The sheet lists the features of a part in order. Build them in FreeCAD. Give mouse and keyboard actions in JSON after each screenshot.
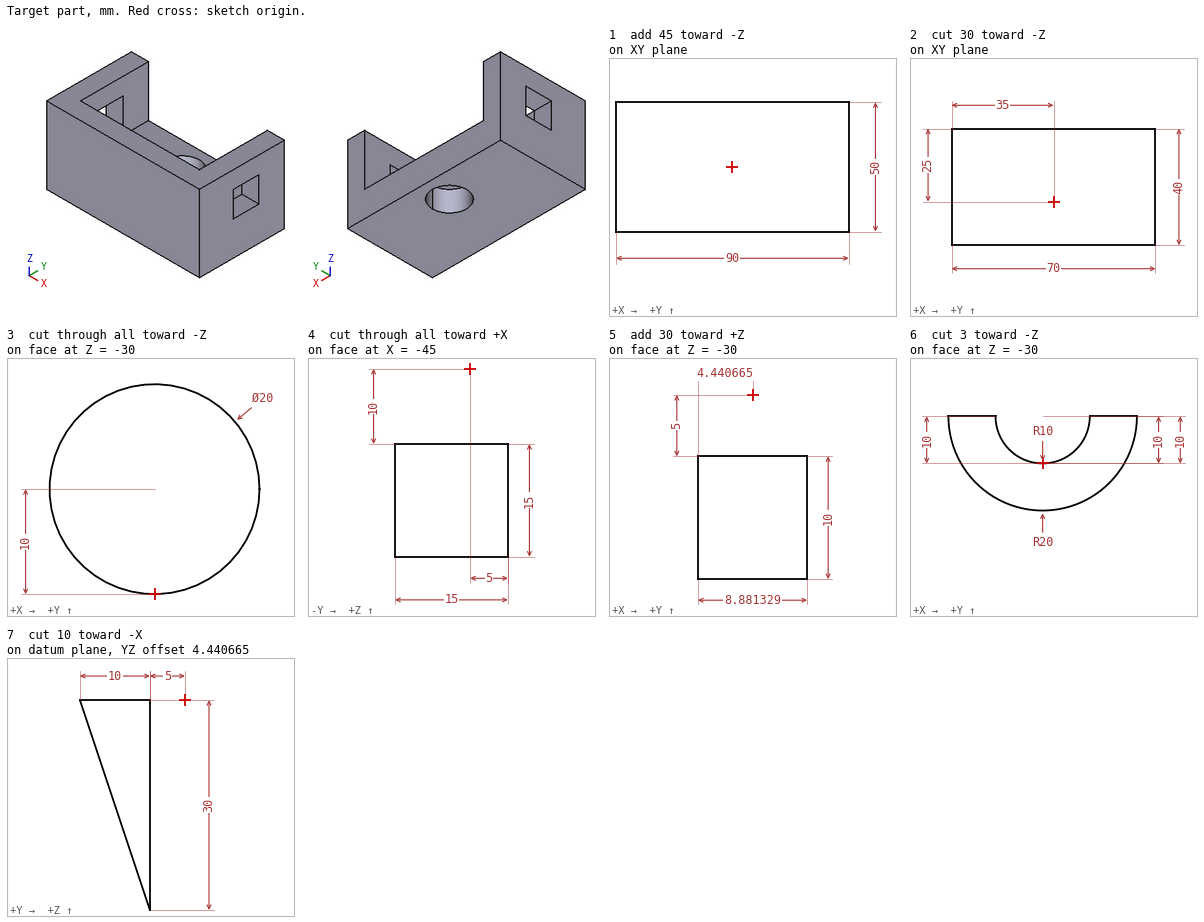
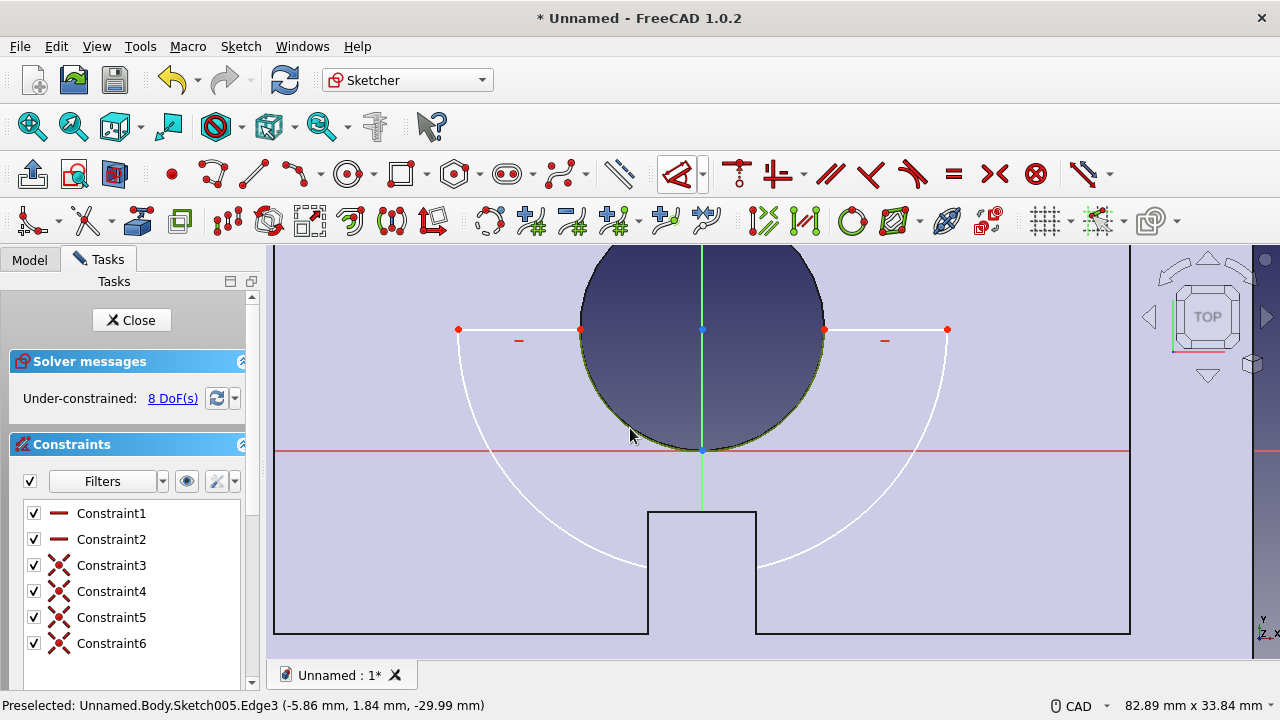
{"action": "left_click", "coordinate": [559, 527]}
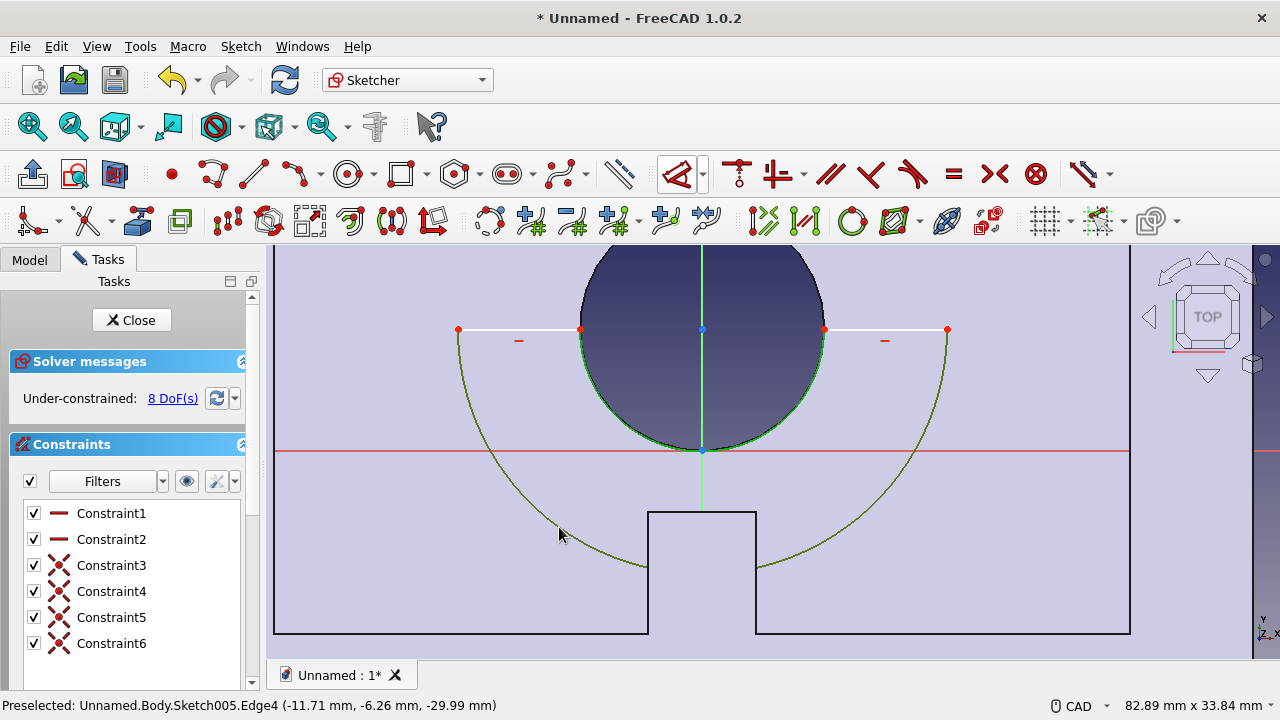
{"action": "key", "text": "c"}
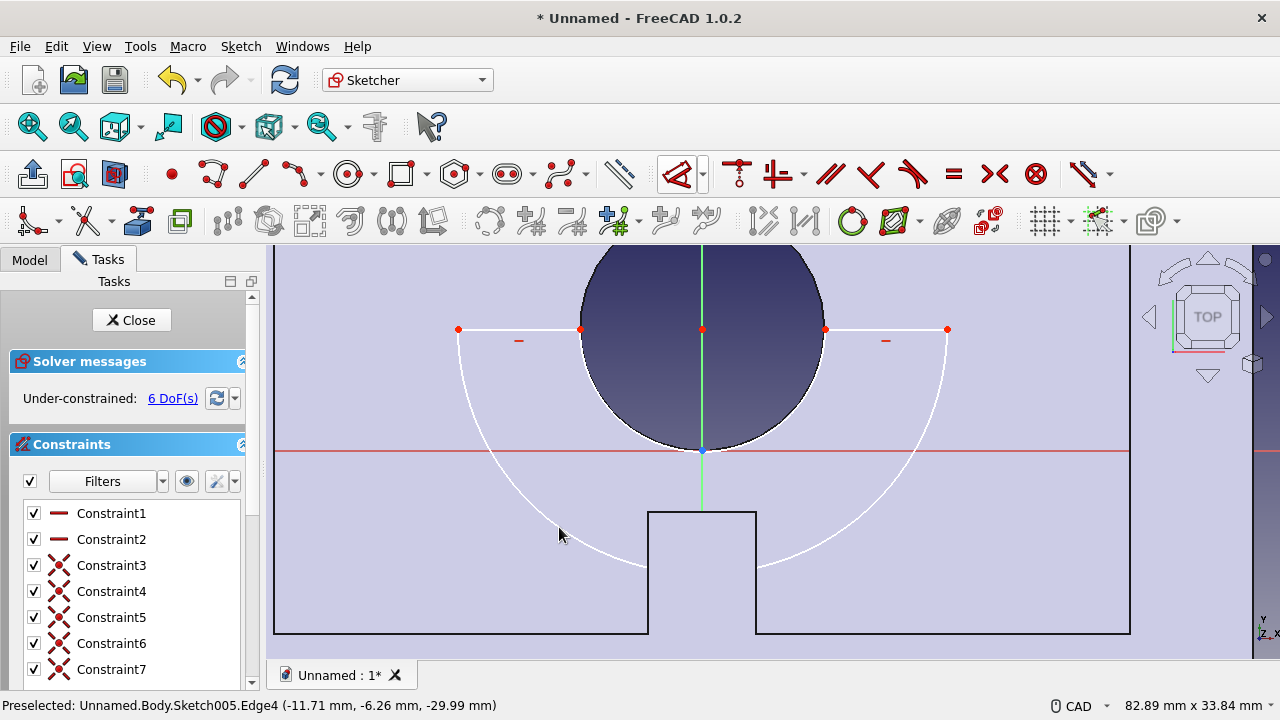
{"action": "left_click", "coordinate": [703, 329]}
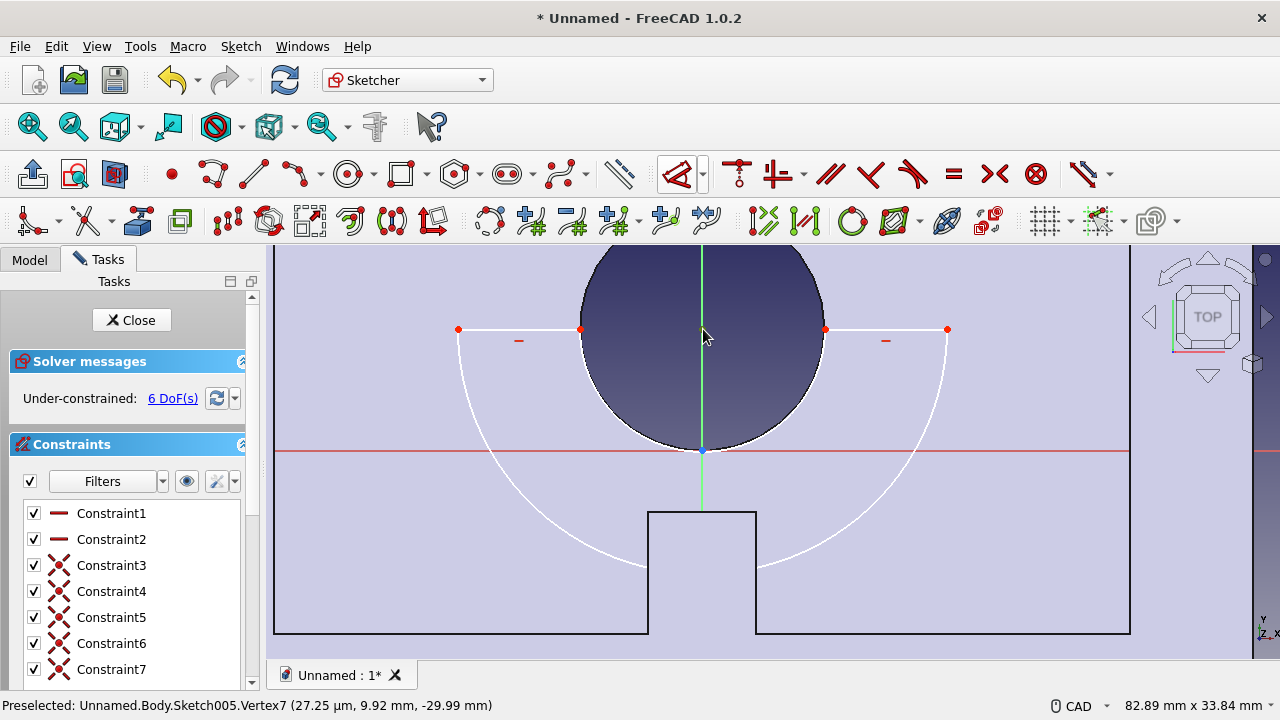
{"action": "left_click", "coordinate": [702, 605]}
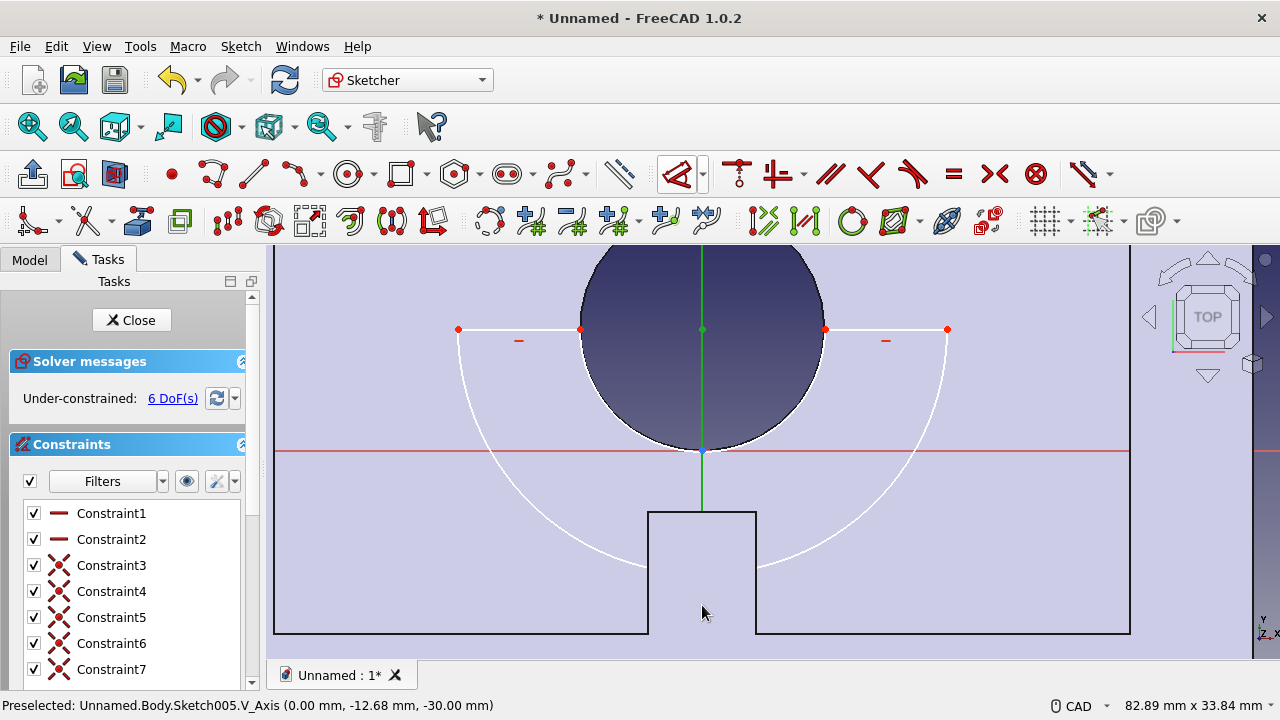
{"action": "key", "text": "c"}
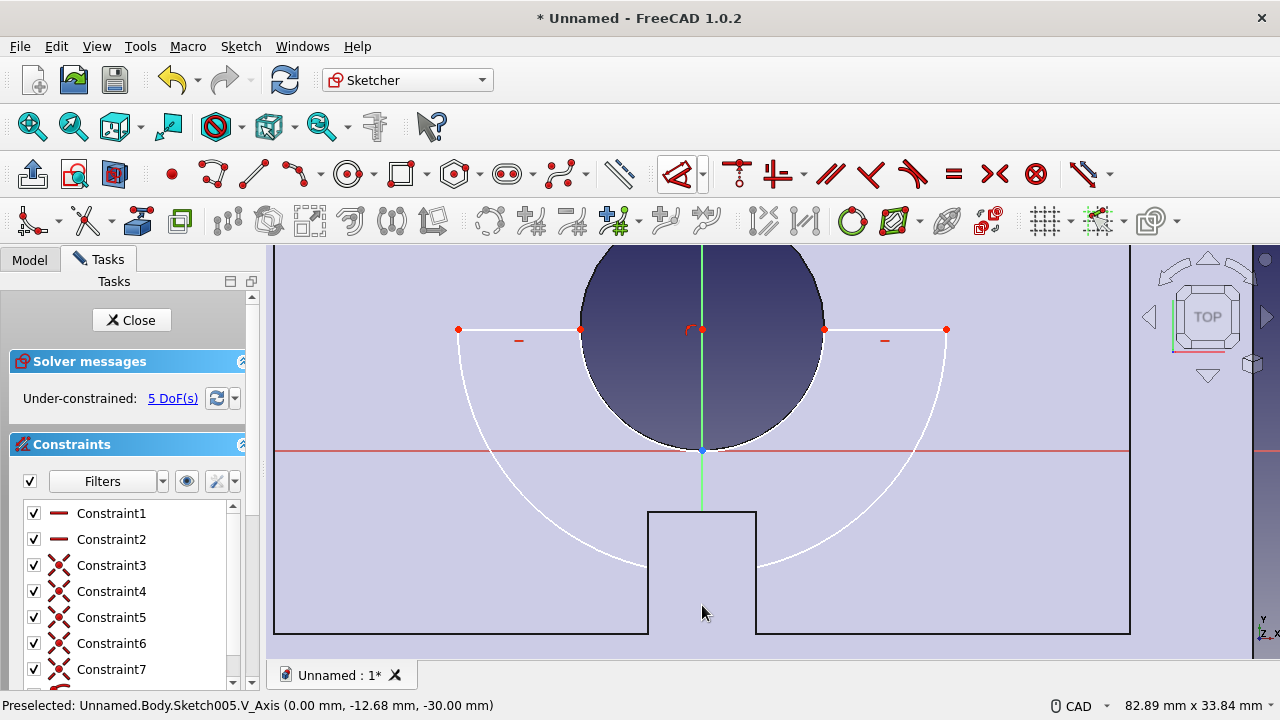
{"action": "left_click", "coordinate": [631, 428]}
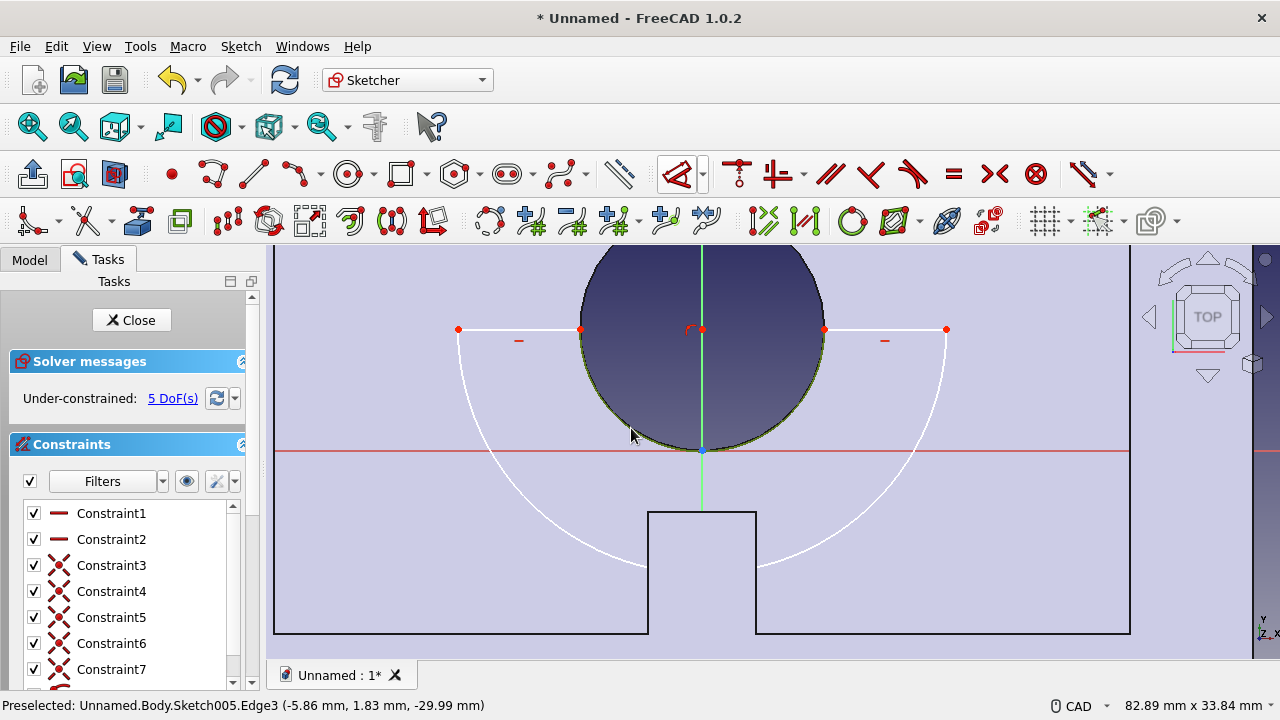
{"action": "key", "text": "k r"}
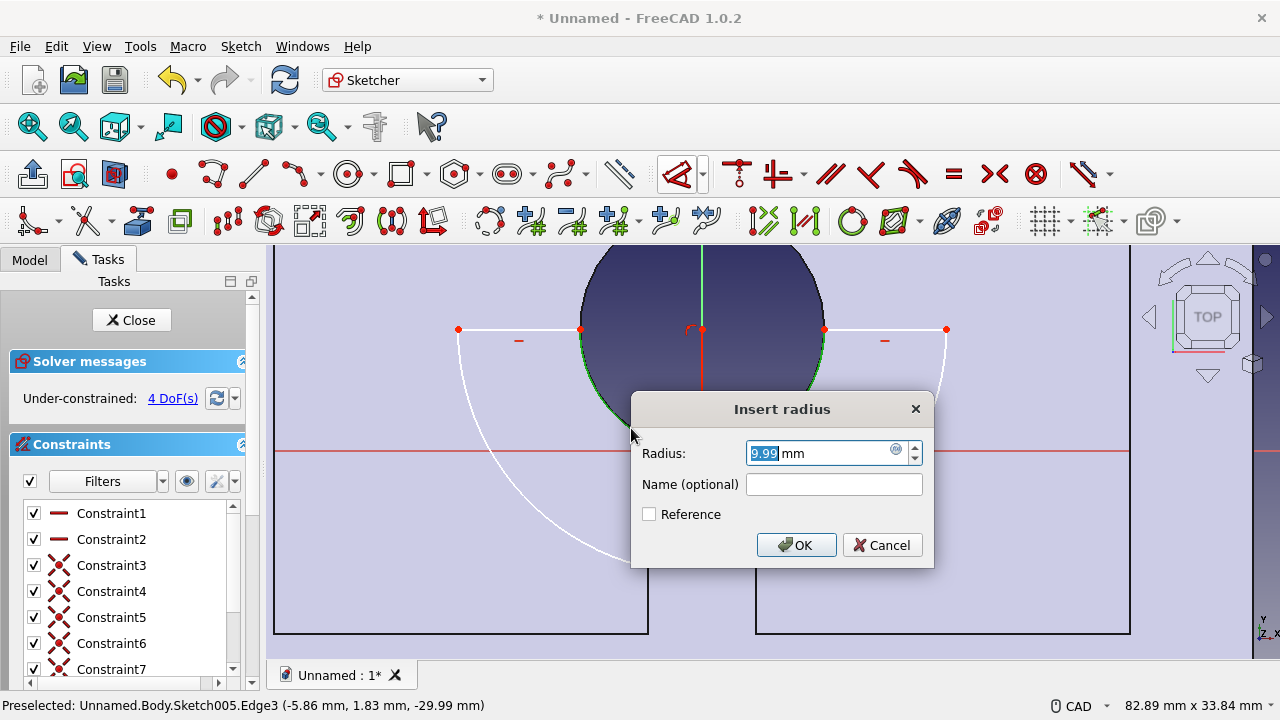
{"action": "type", "text": "10"}
{"action": "key", "text": "Return"}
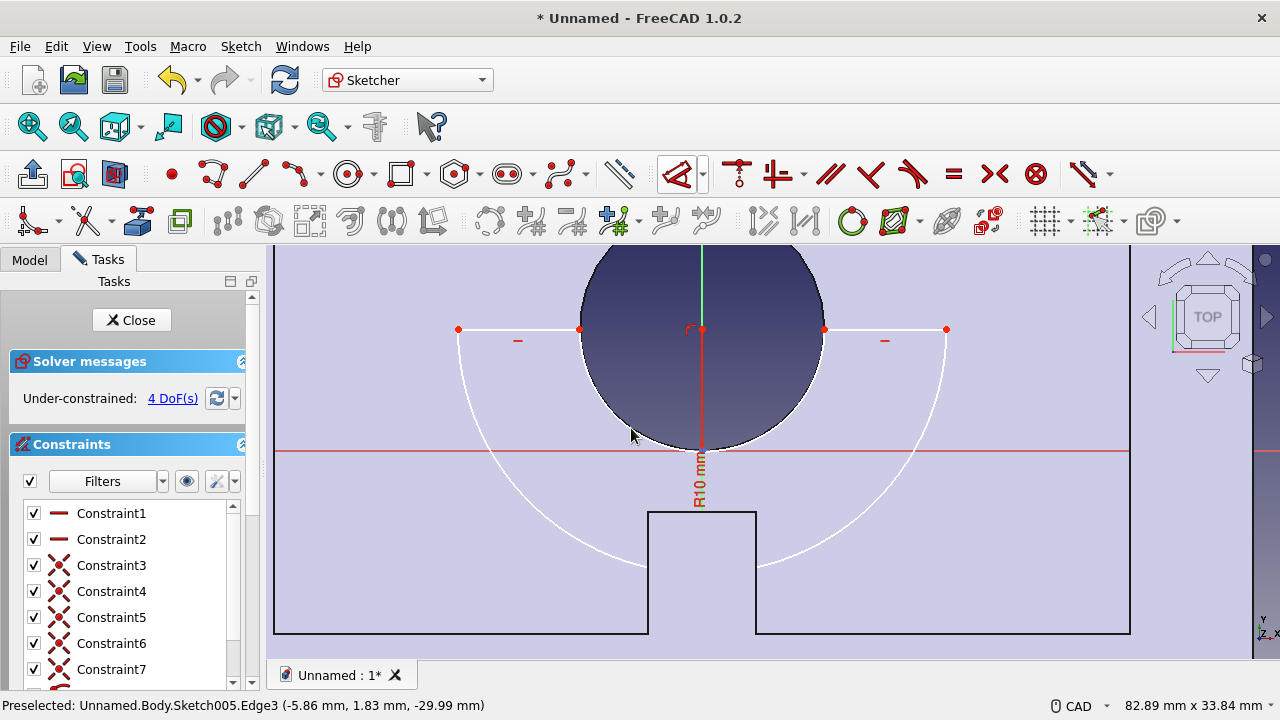
{"action": "left_click", "coordinate": [559, 527]}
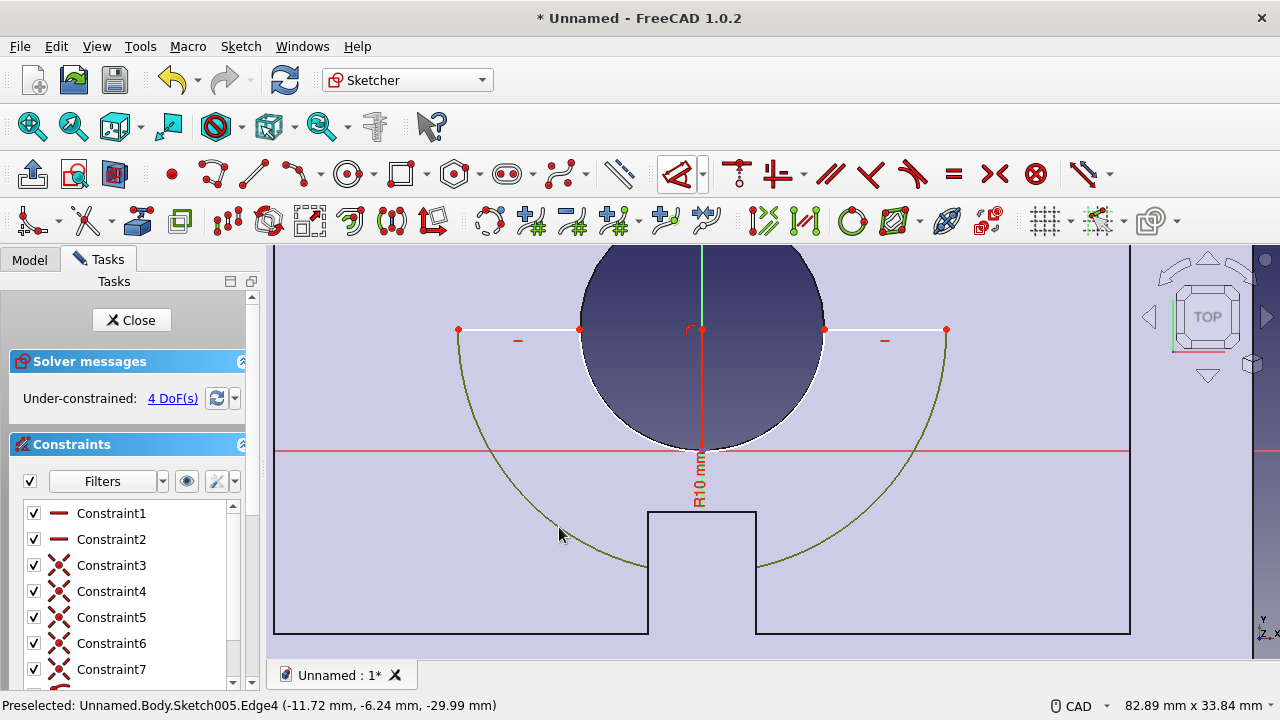
{"action": "key", "text": "k r"}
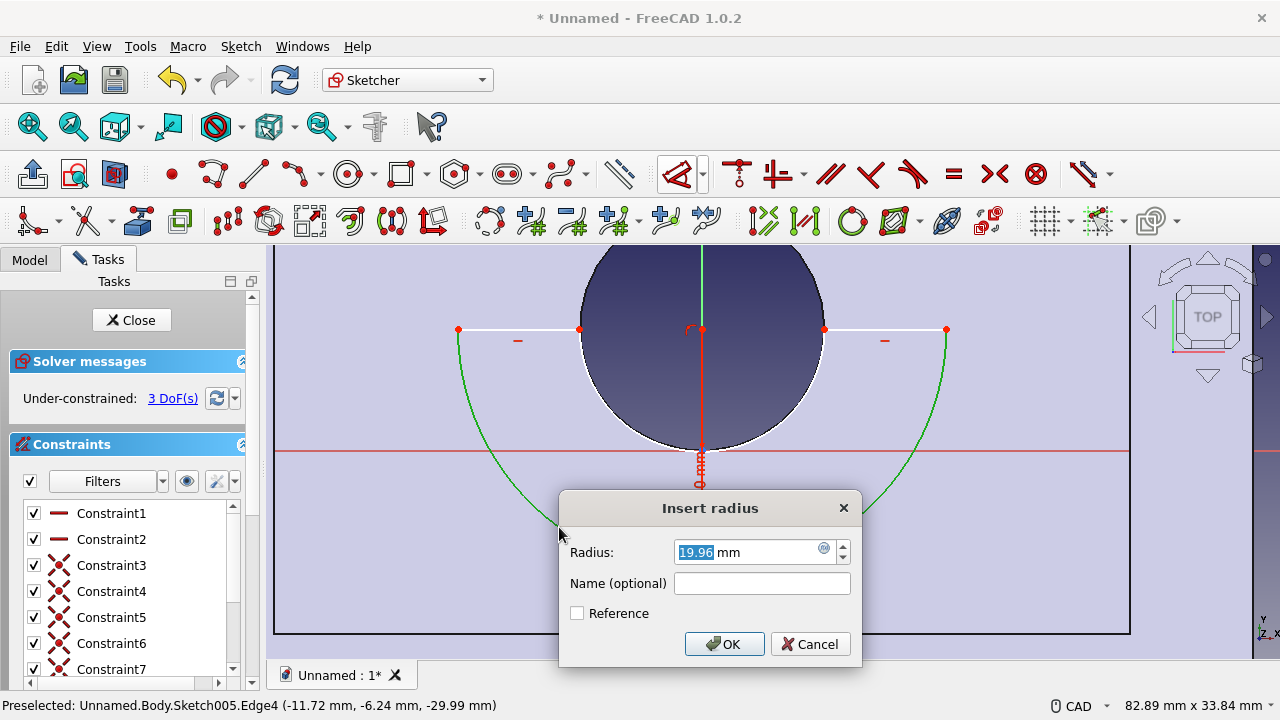
{"action": "type", "text": "20"}
{"action": "key", "text": "Return"}